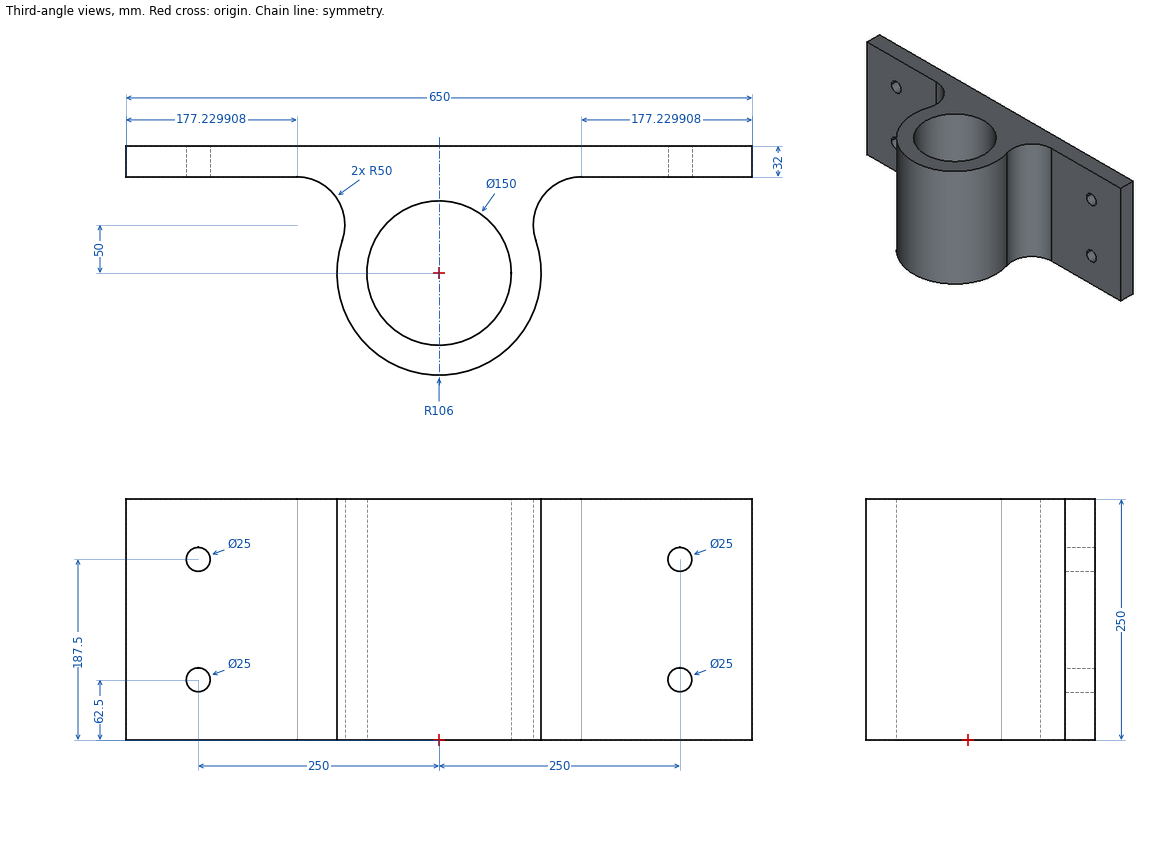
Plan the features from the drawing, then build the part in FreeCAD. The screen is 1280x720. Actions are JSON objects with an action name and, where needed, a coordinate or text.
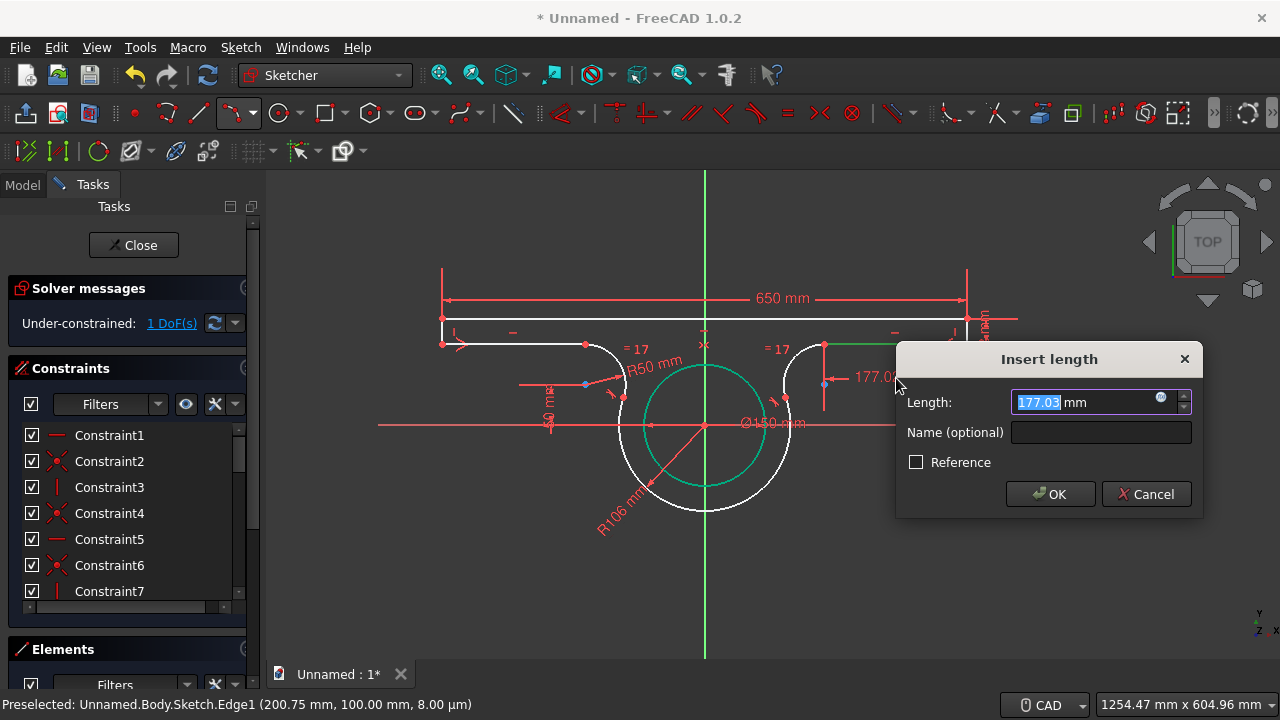
{"action": "type", "text": "177.229908"}
{"action": "key", "text": "Return"}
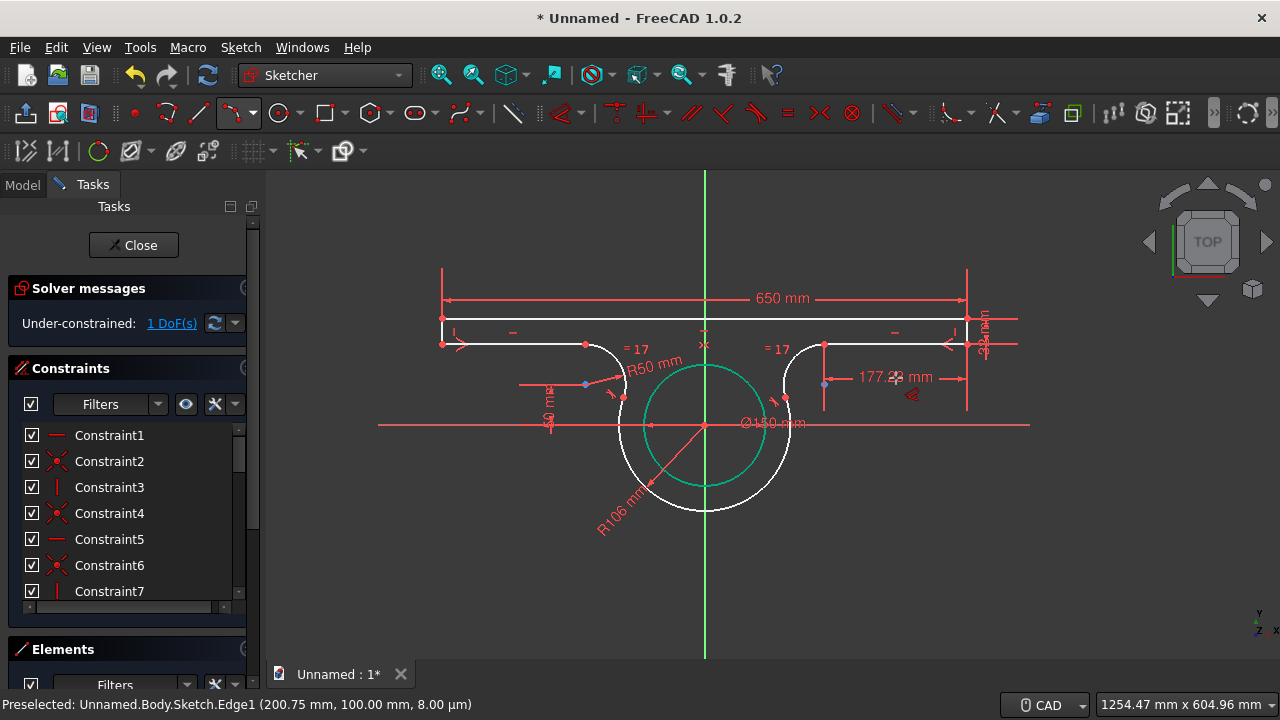
{"action": "left_click", "coordinate": [485, 344]}
{"action": "left_click", "coordinate": [514, 378]}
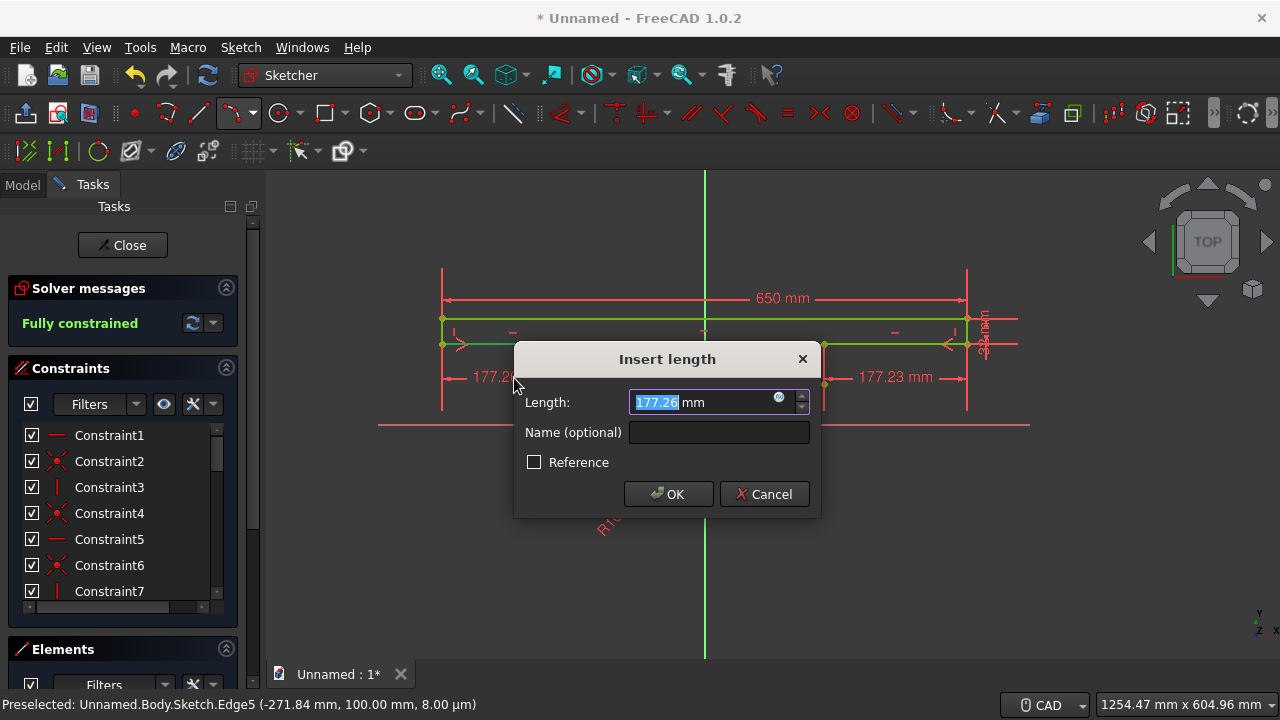
{"action": "type", "text": "177.229908"}
{"action": "key", "text": "Return"}
{"action": "key", "text": "Escape"}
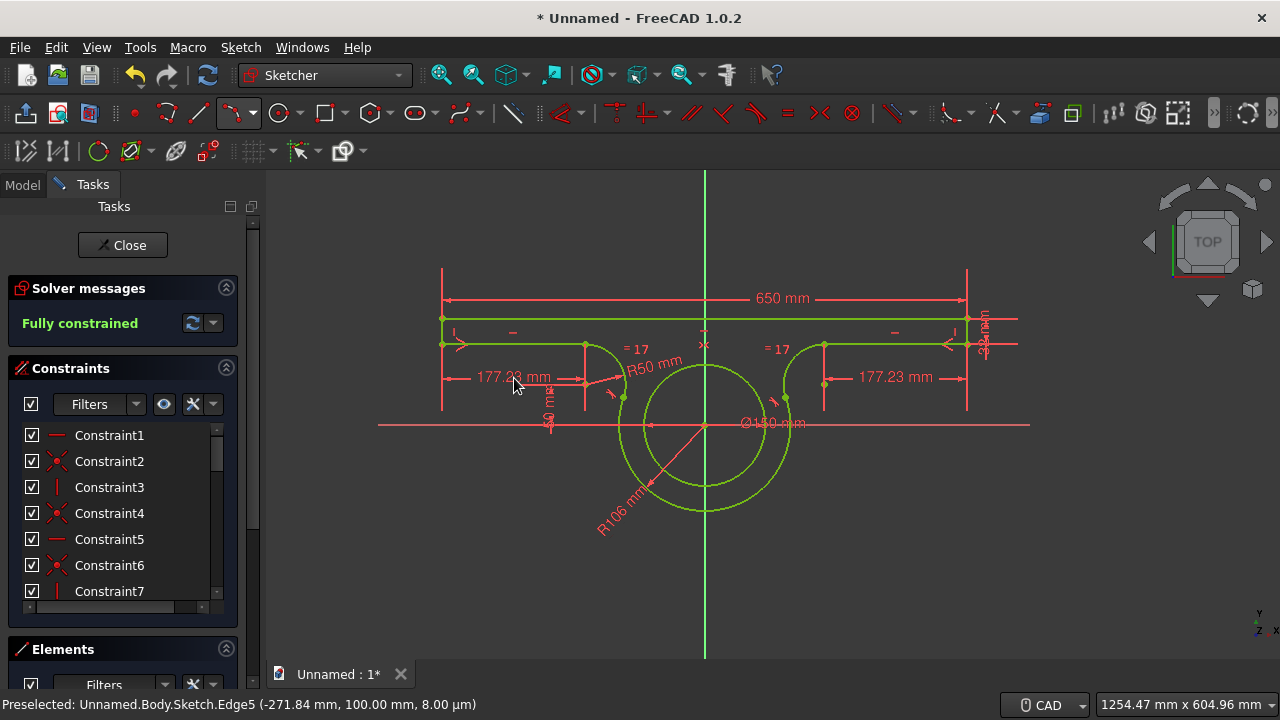
{"action": "left_click", "coordinate": [123, 245]}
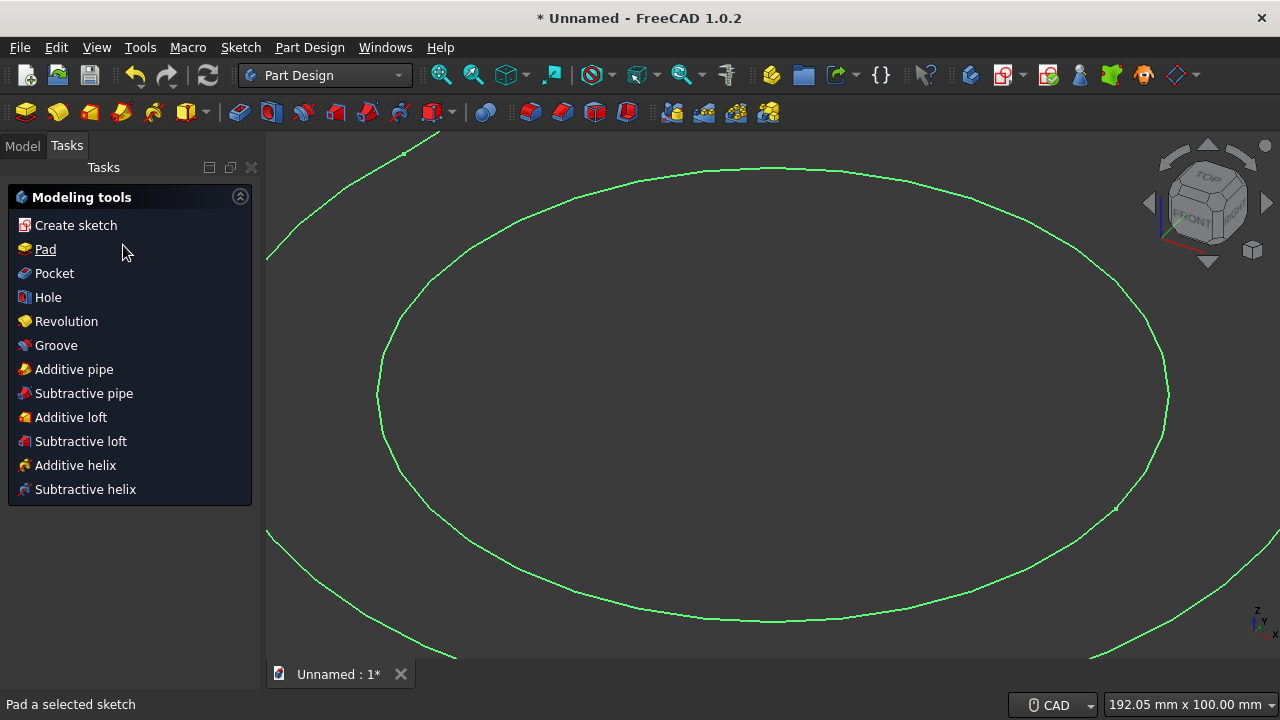
{"action": "left_click", "coordinate": [26, 112]}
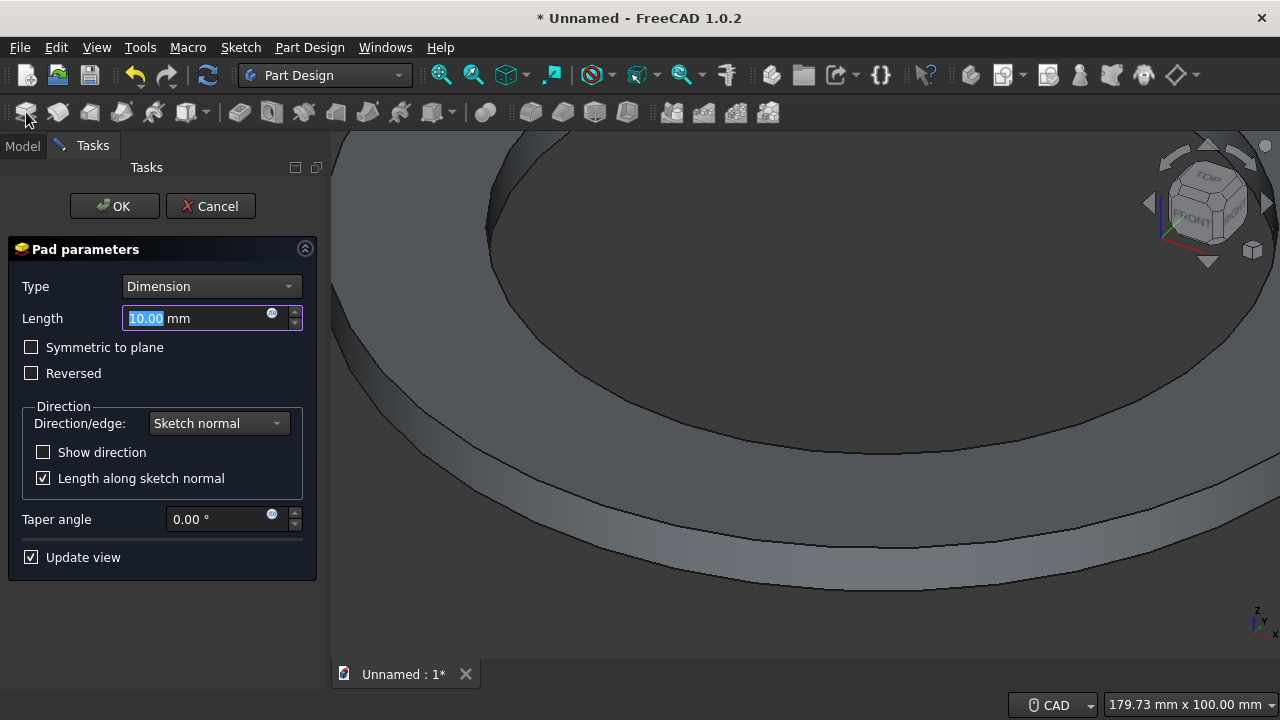
{"action": "type", "text": "250"}
{"action": "key", "text": "Tab"}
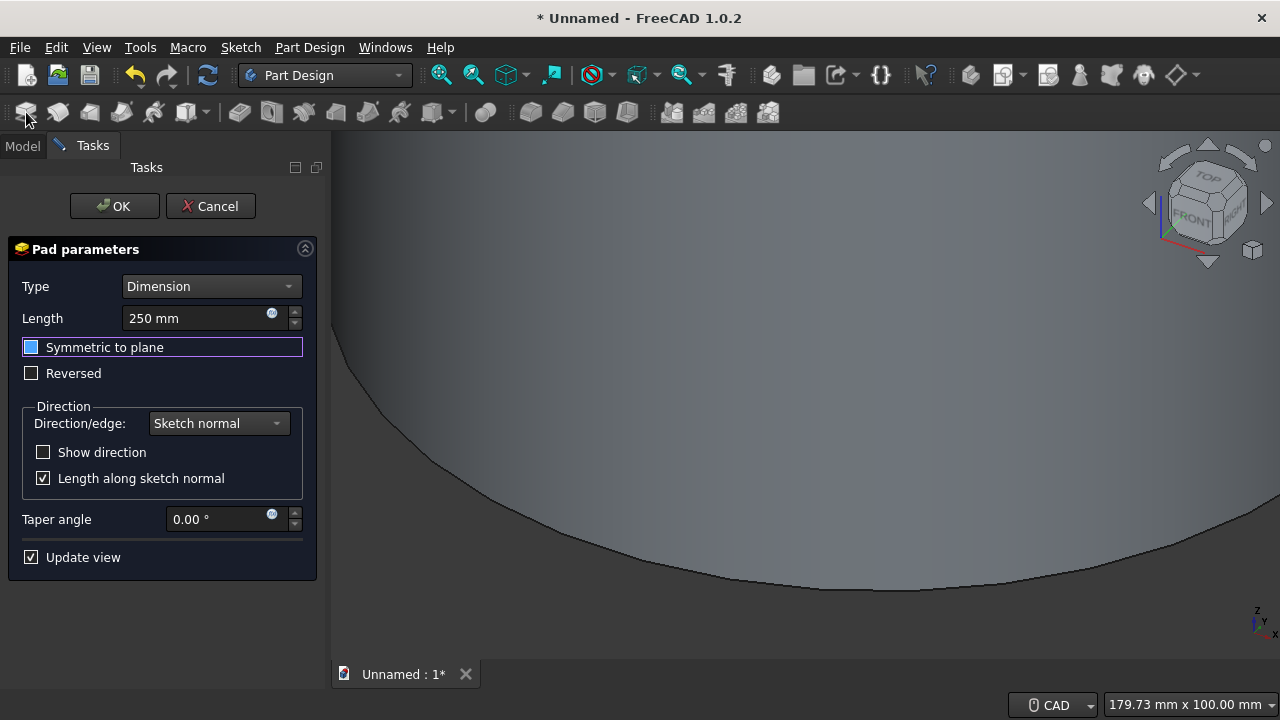
{"action": "left_click", "coordinate": [115, 206]}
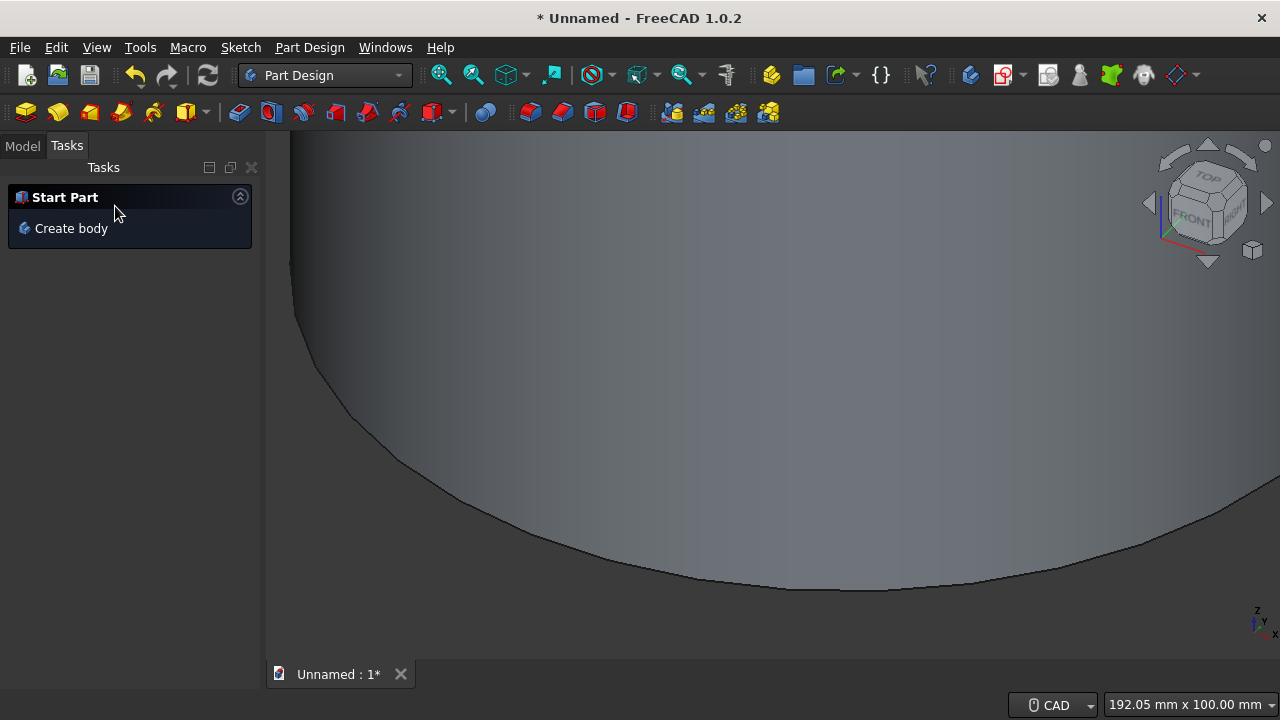
{"action": "left_click", "coordinate": [442, 76]}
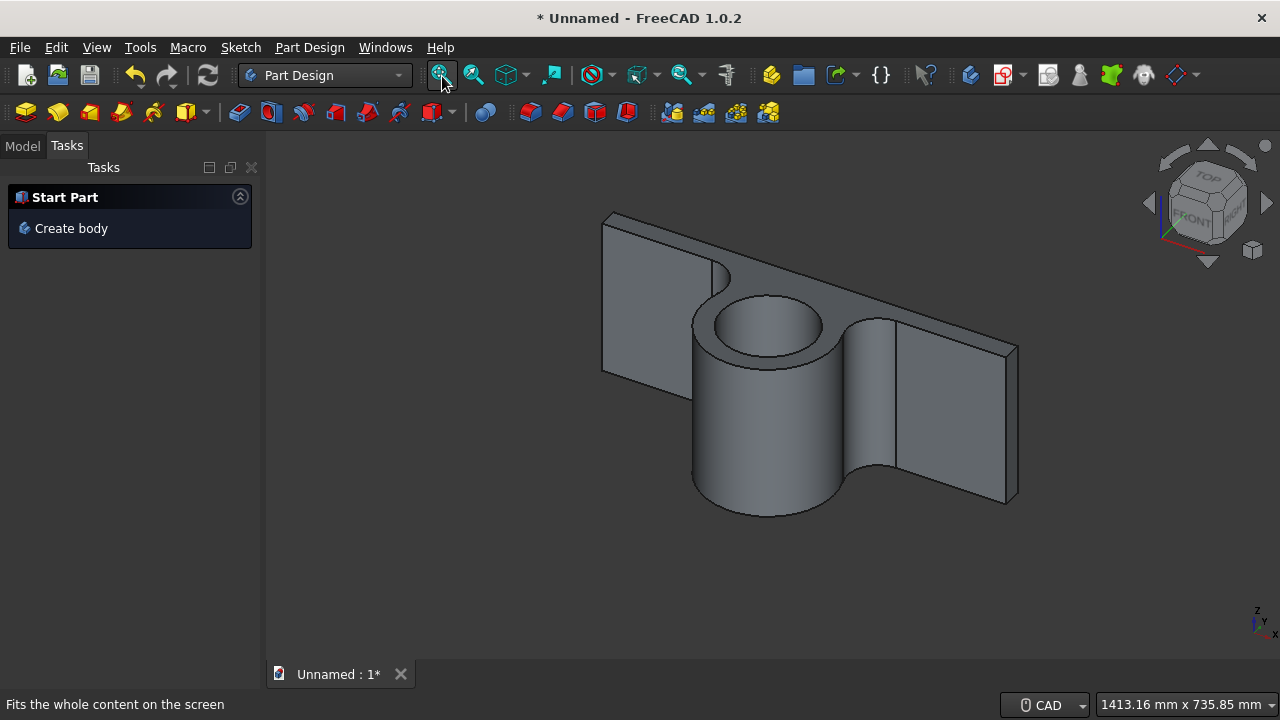
{"action": "key", "text": "4"}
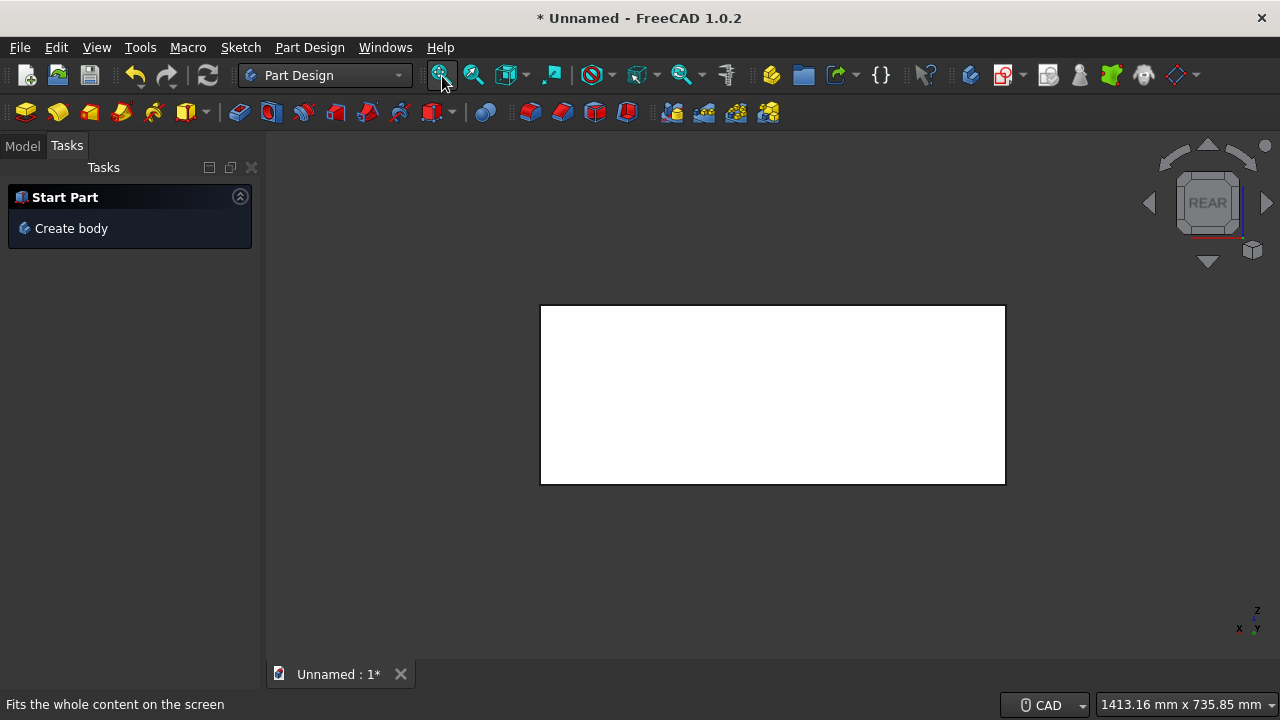
{"action": "left_click", "coordinate": [640, 394]}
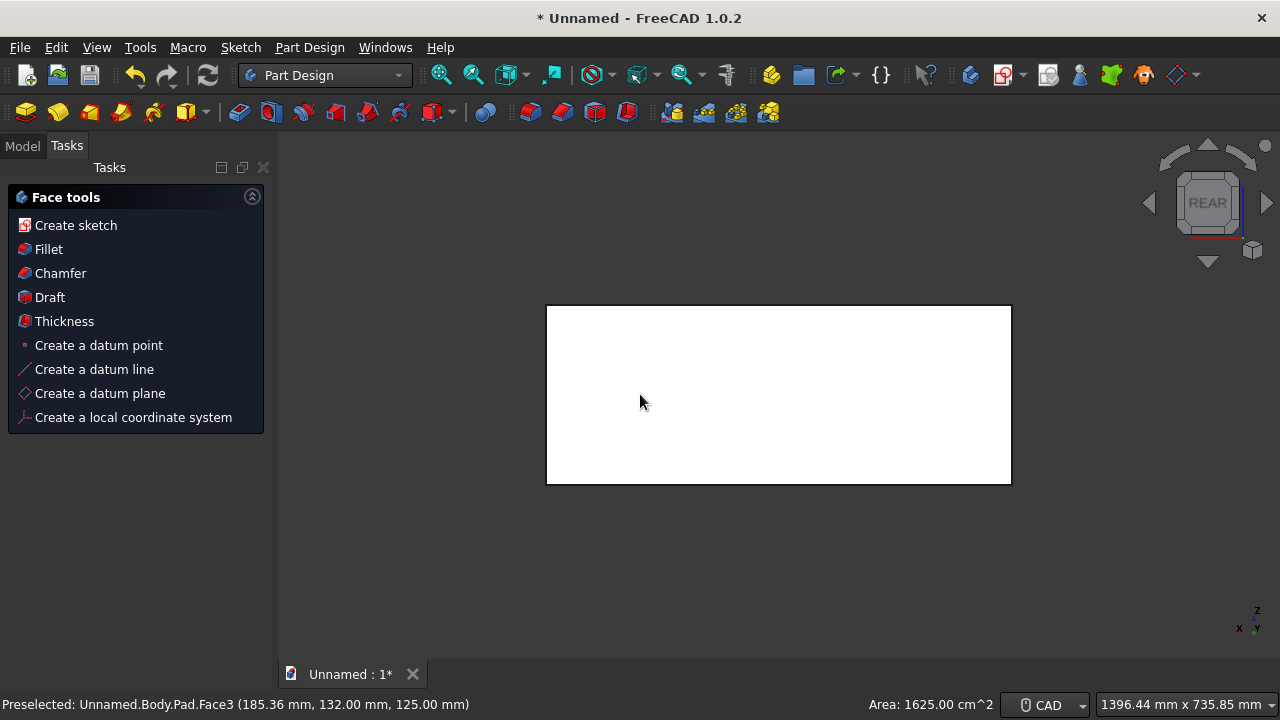
{"action": "left_click", "coordinate": [1004, 76]}